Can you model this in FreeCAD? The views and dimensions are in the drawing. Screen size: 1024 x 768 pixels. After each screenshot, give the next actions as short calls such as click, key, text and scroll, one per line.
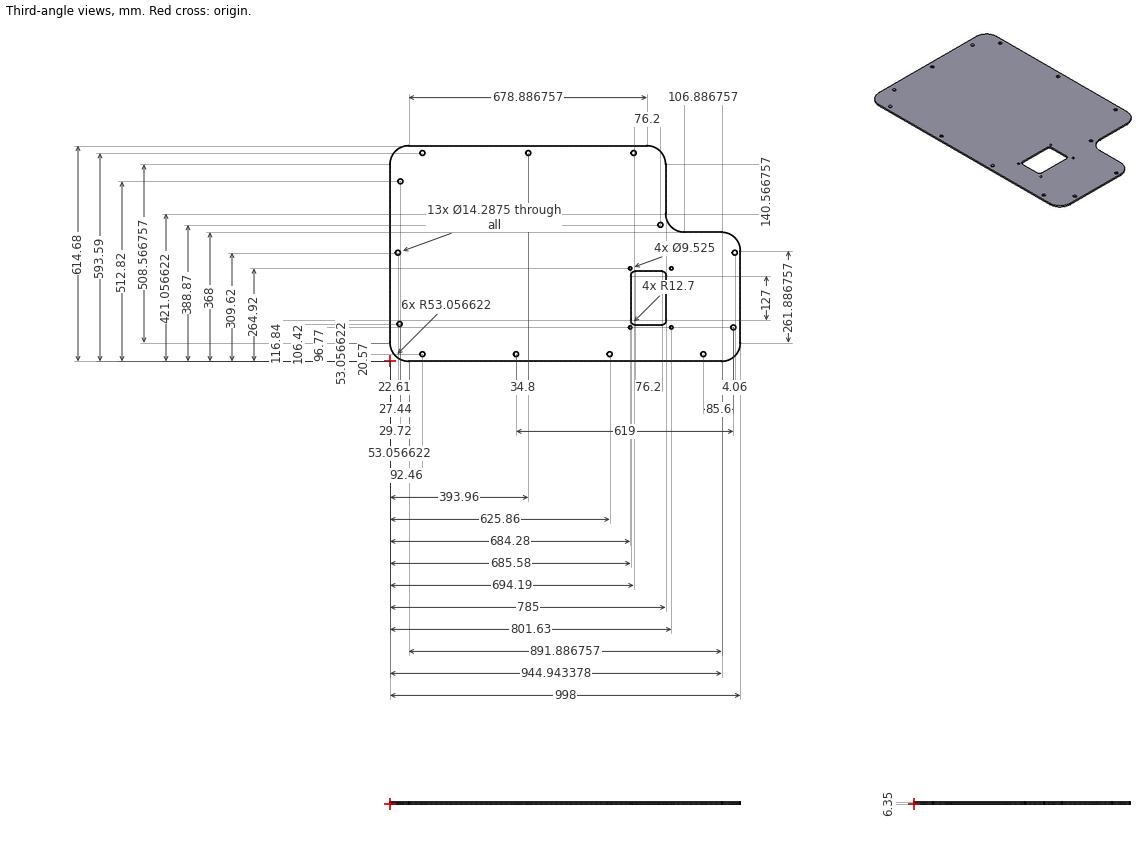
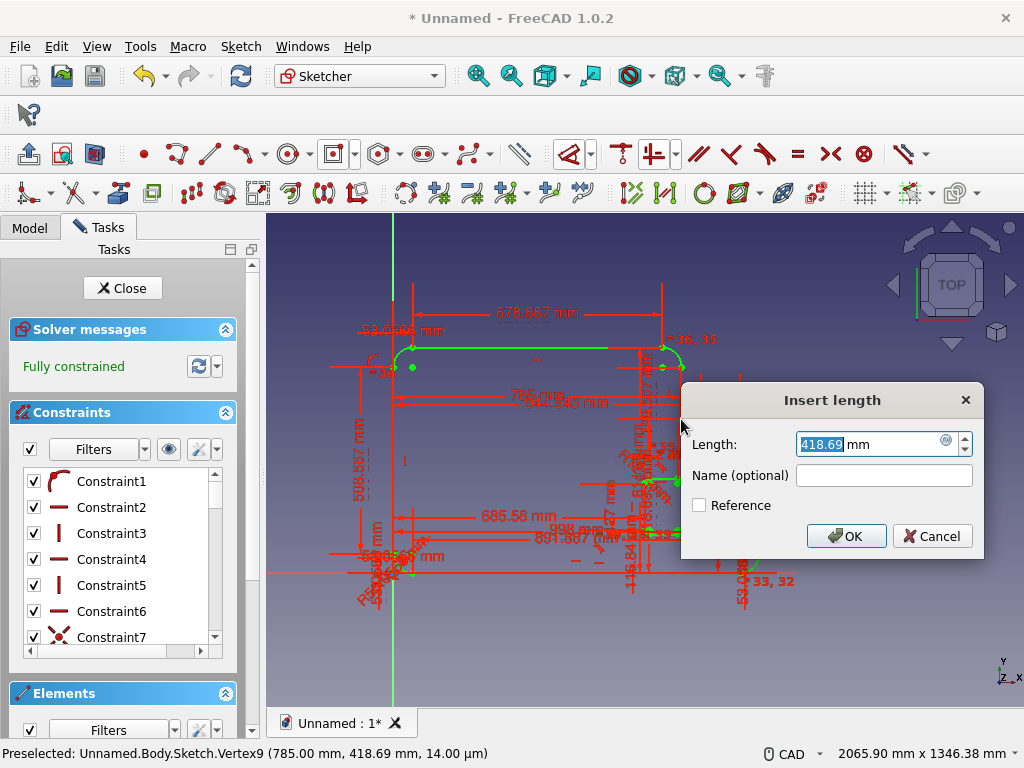
text(421.056622)
key(Return)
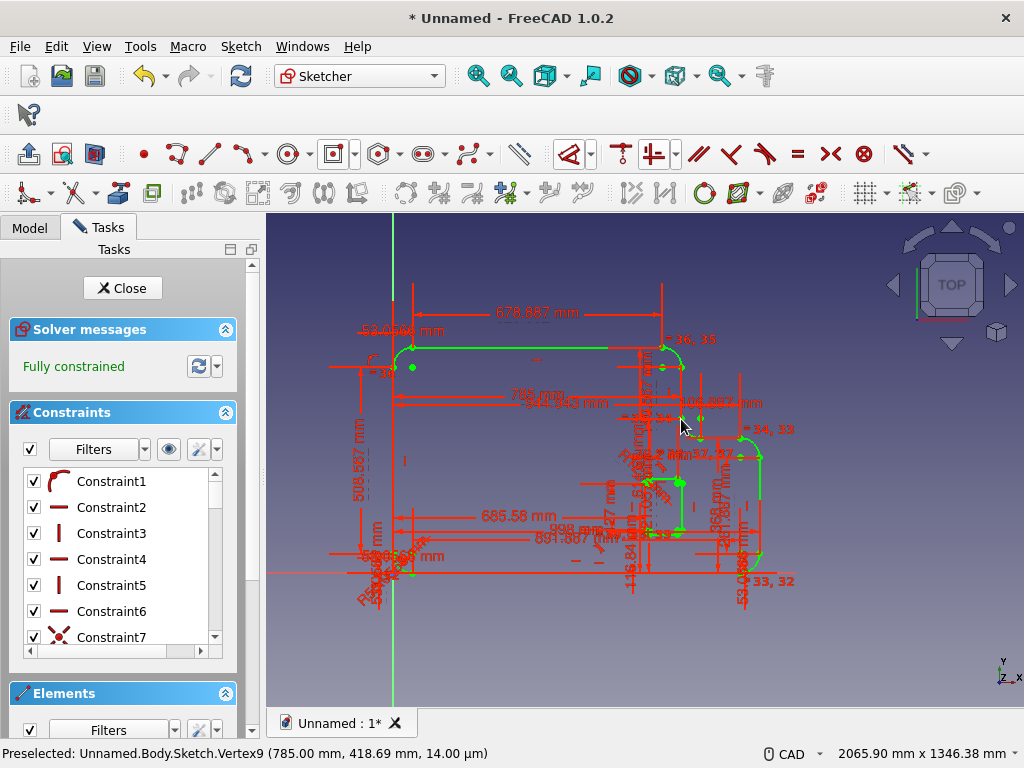
click(123, 288)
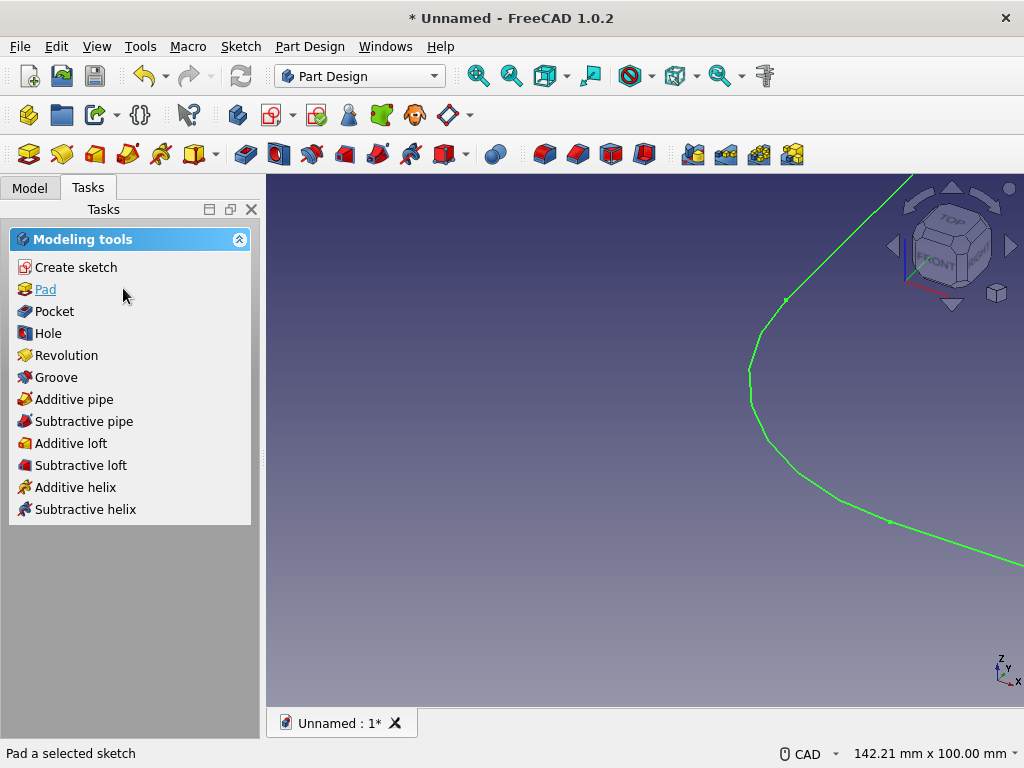
click(29, 154)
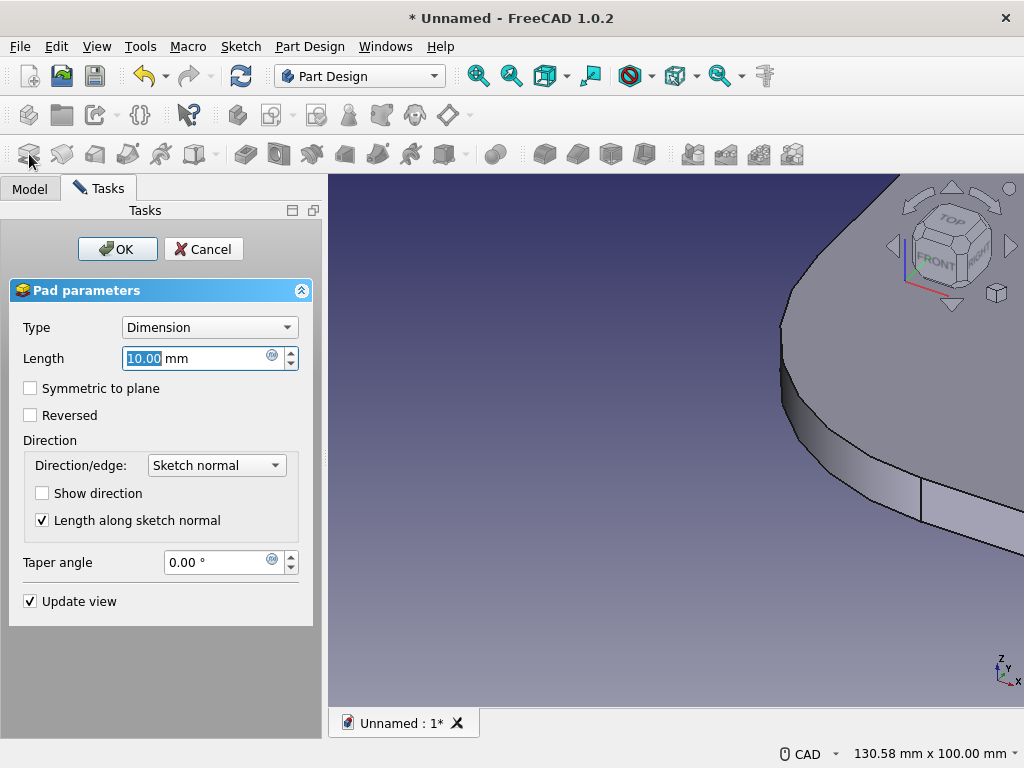
text(6.35)
key(Tab)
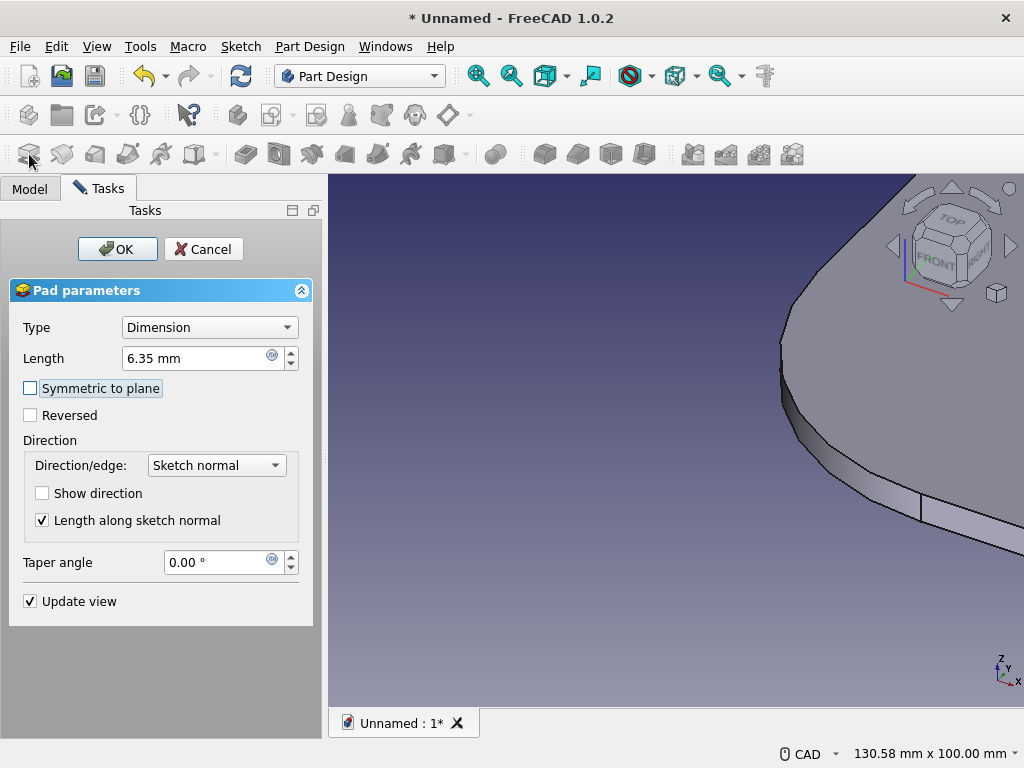
click(118, 249)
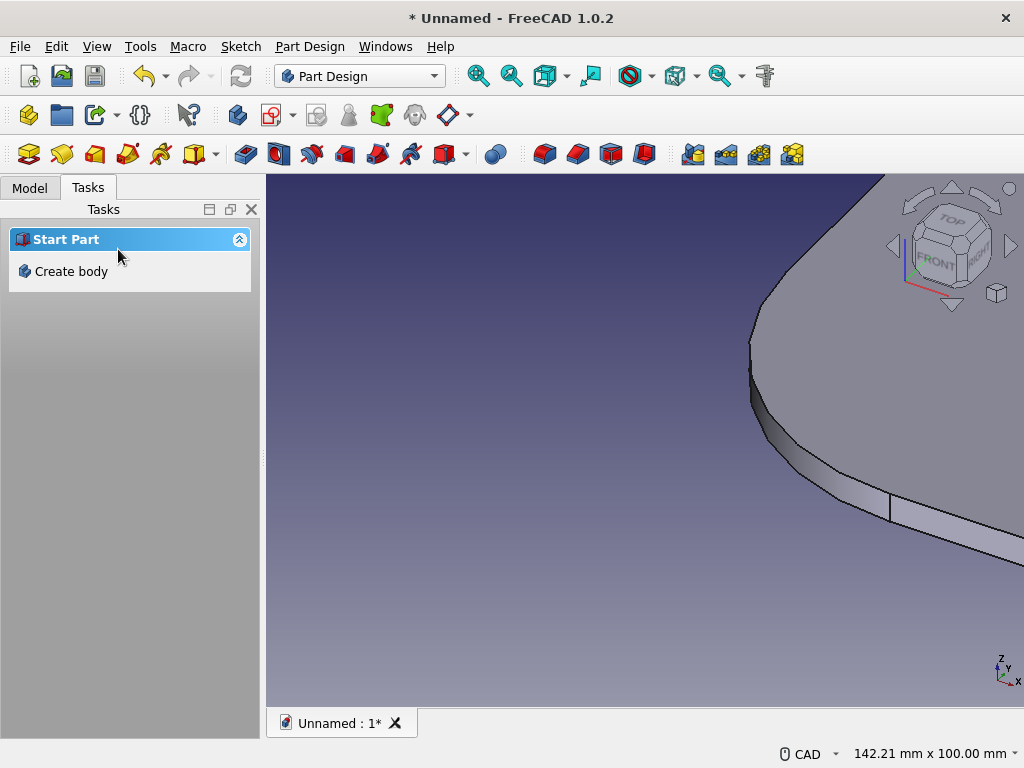
click(479, 76)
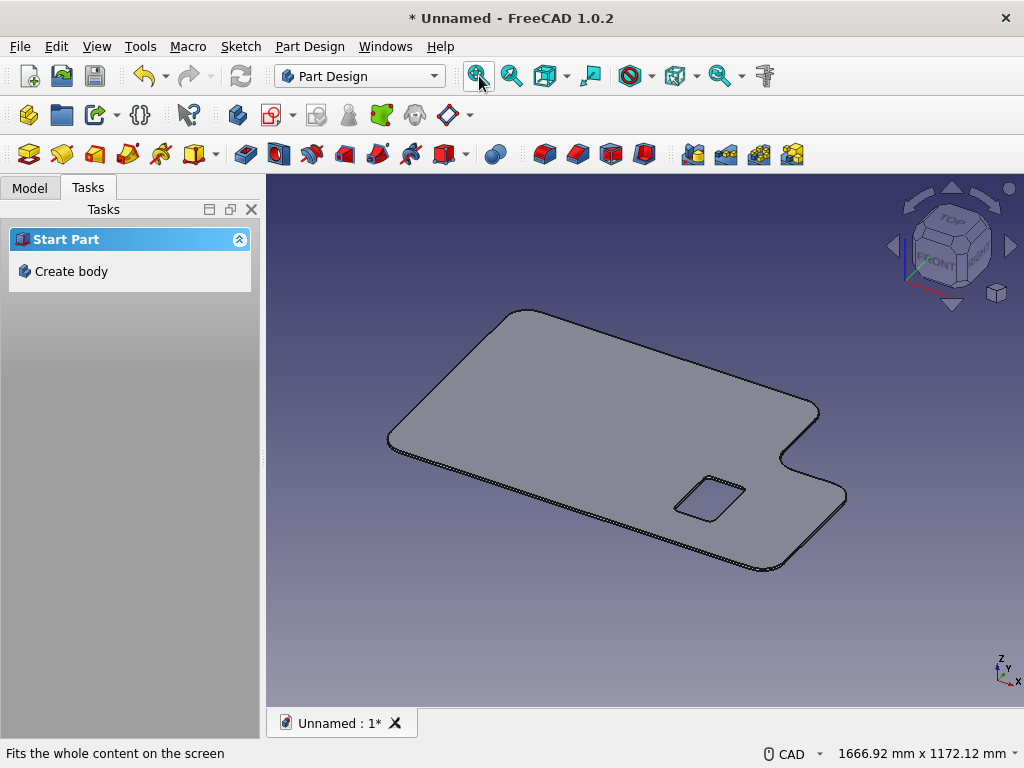
click(589, 420)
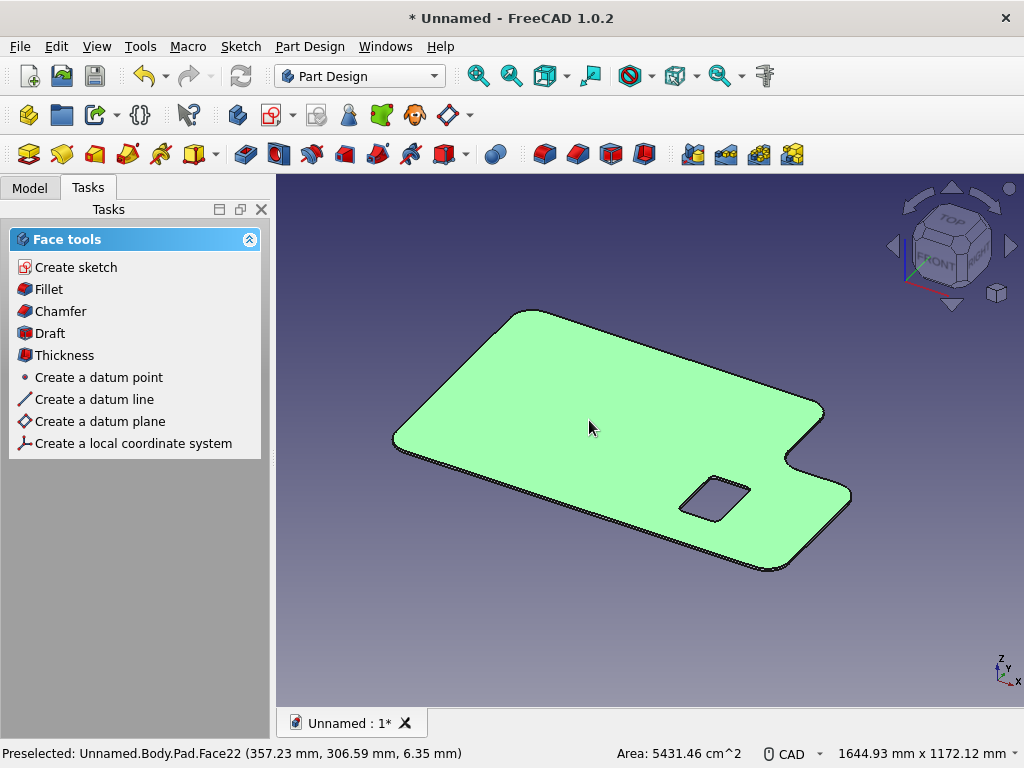
click(270, 116)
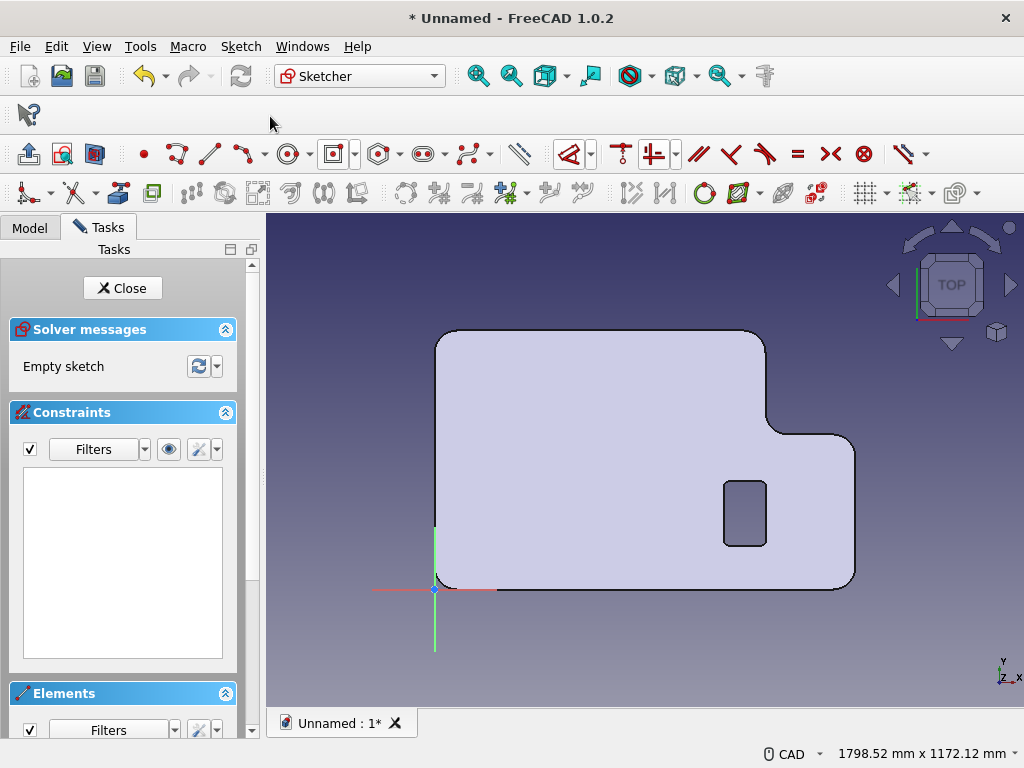
scroll(294, 447, down, 1)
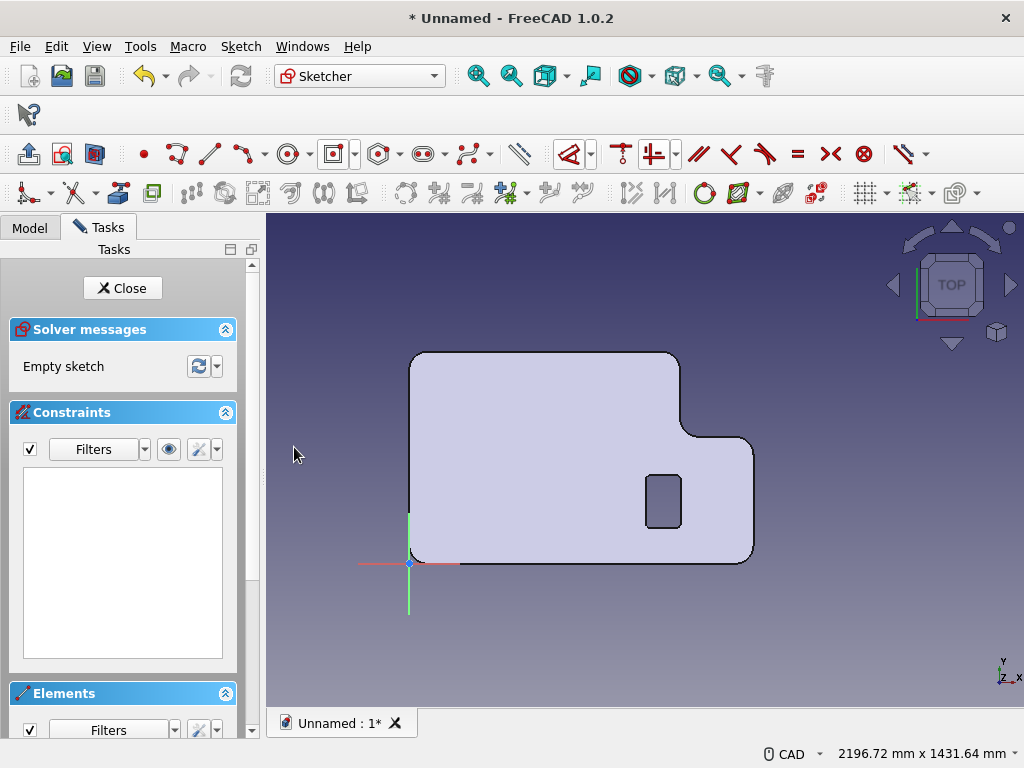
click(288, 154)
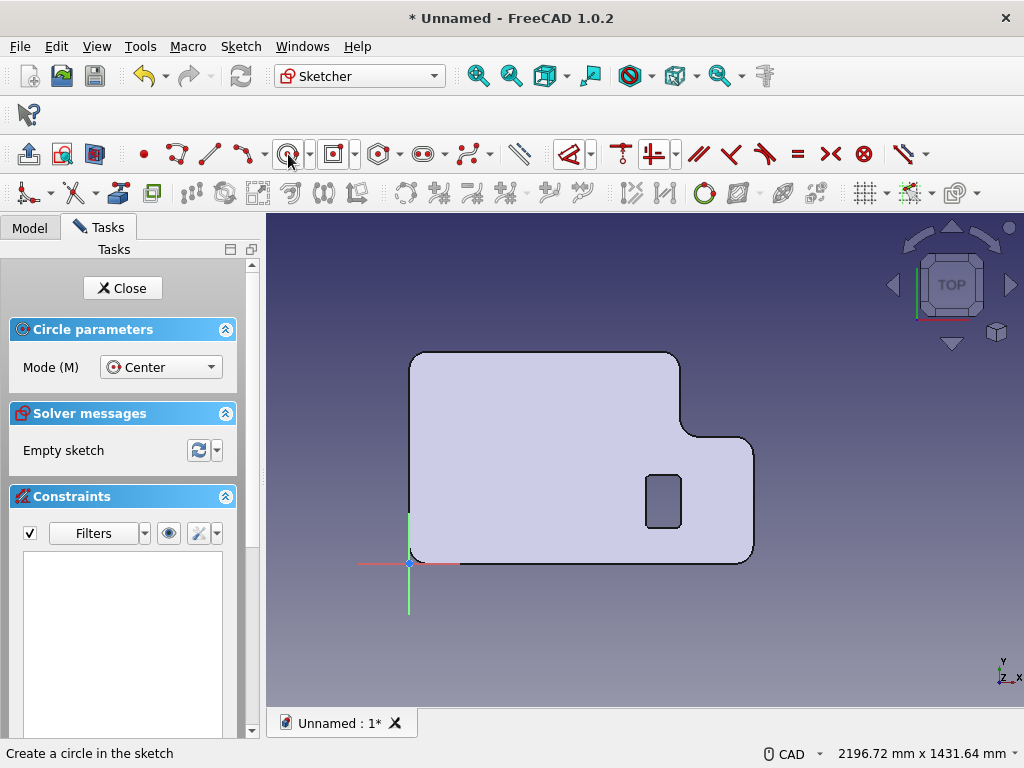
scroll(417, 457, up, 12)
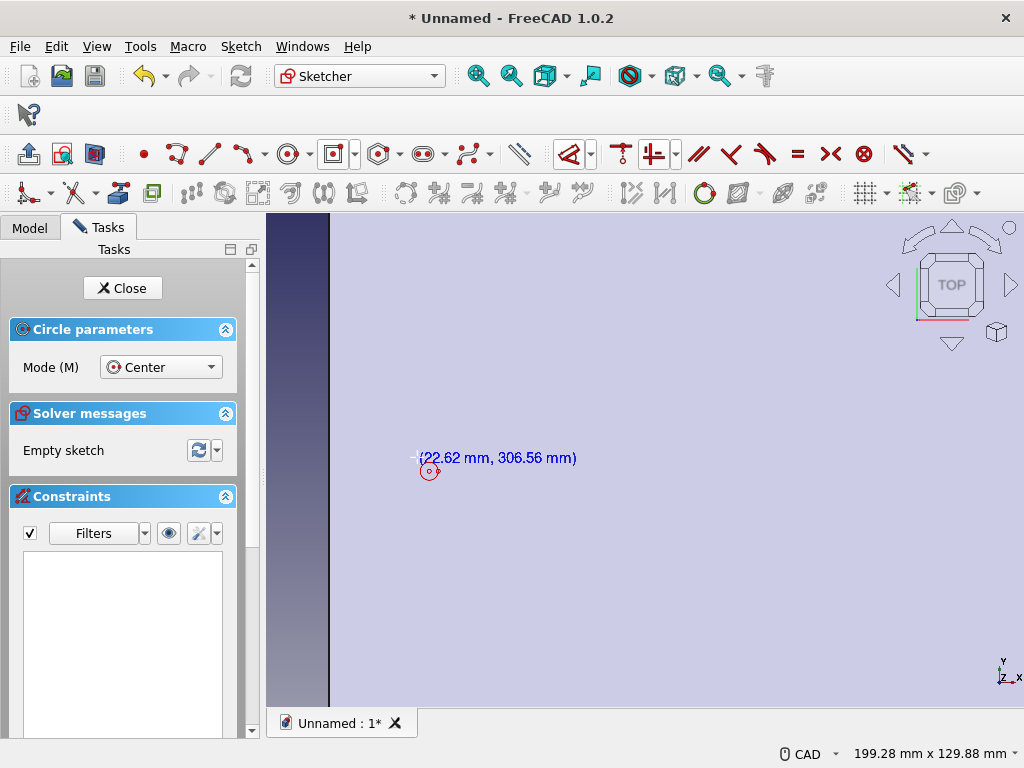
scroll(373, 457, down, 11)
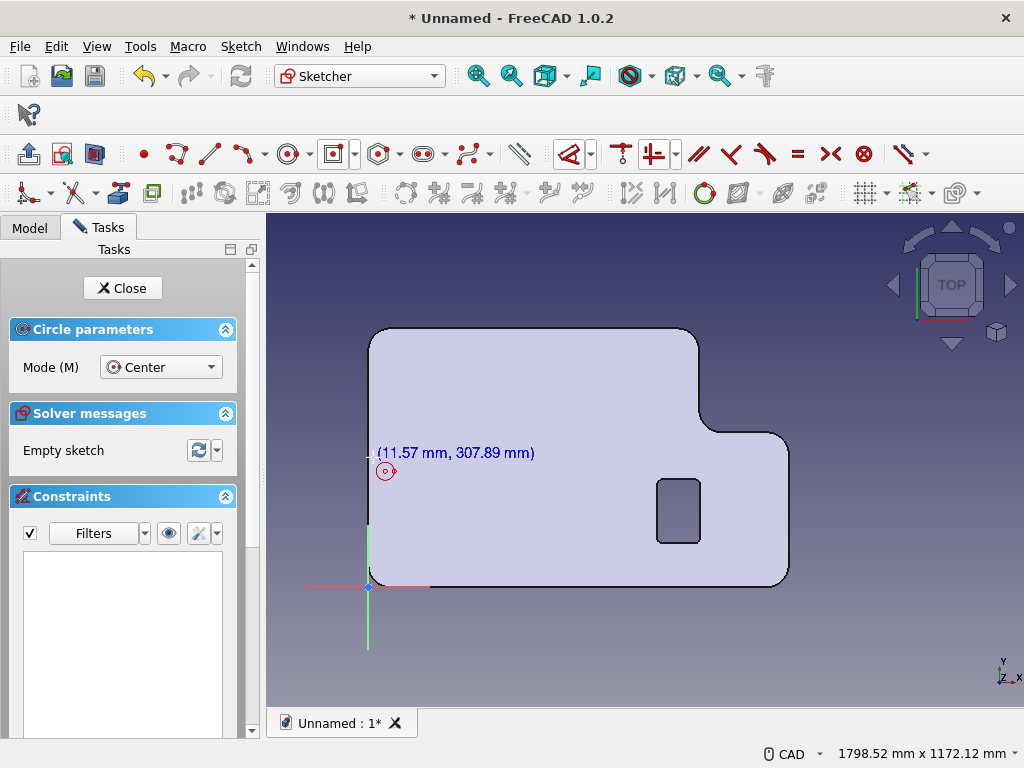
scroll(378, 457, up, 3)